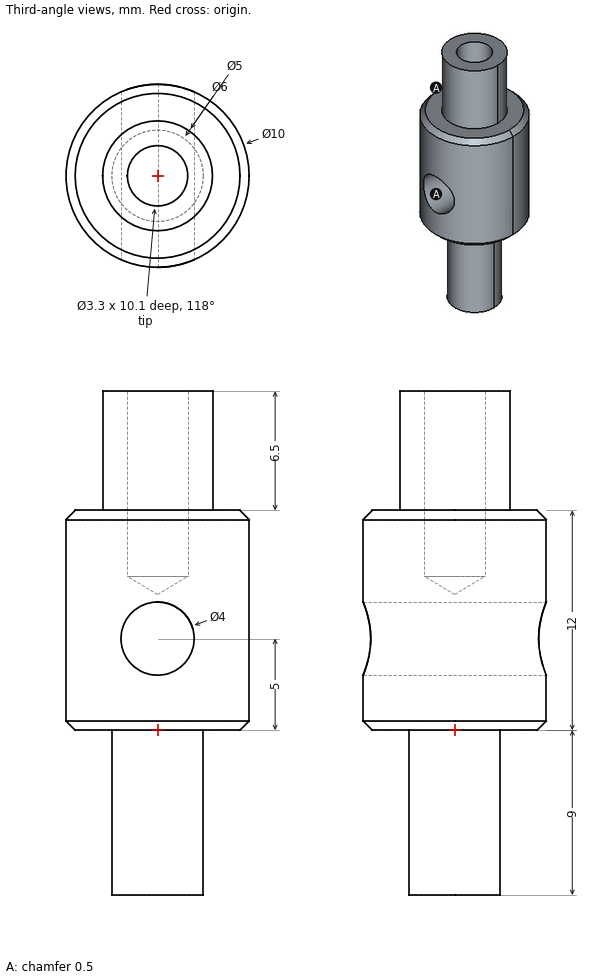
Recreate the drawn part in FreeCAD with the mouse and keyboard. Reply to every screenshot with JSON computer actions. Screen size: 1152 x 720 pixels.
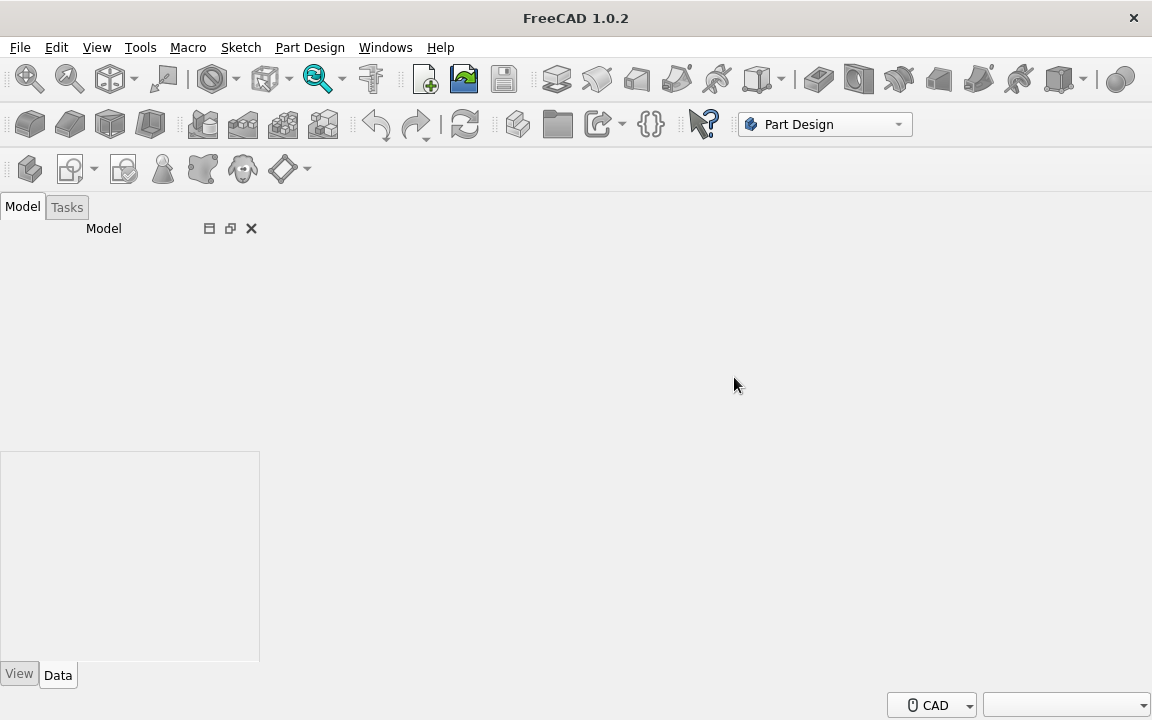
{"action": "key", "text": "ctrl+n"}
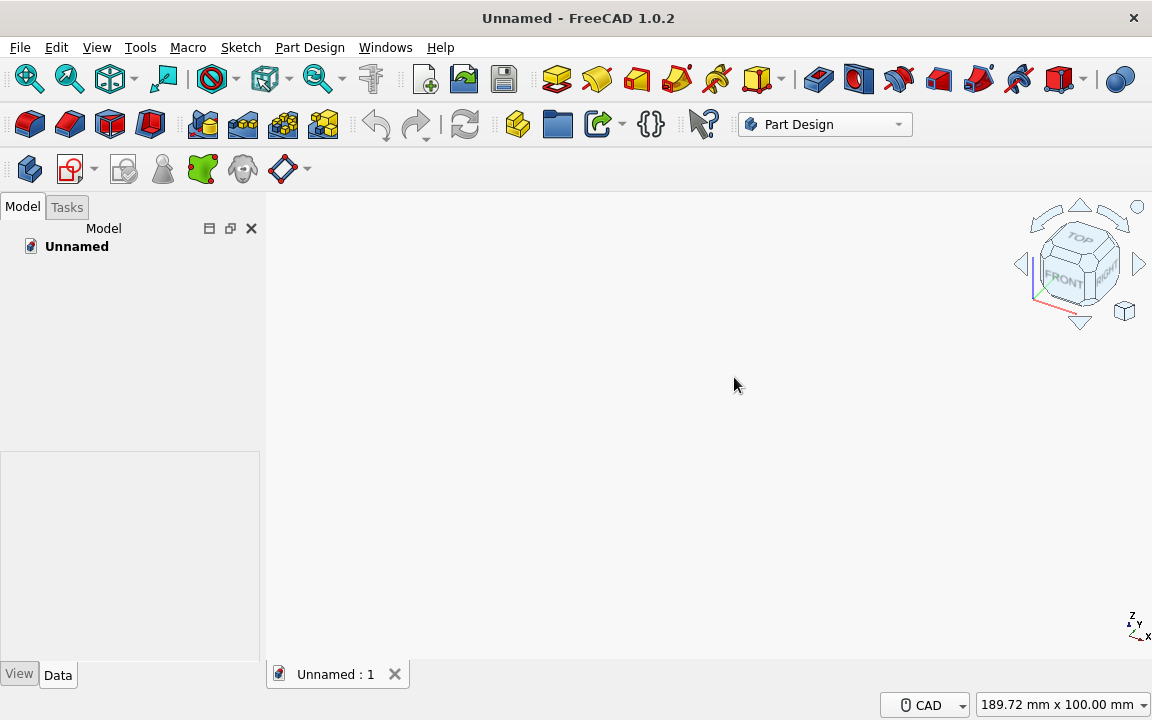
{"action": "left_click", "coordinate": [70, 170]}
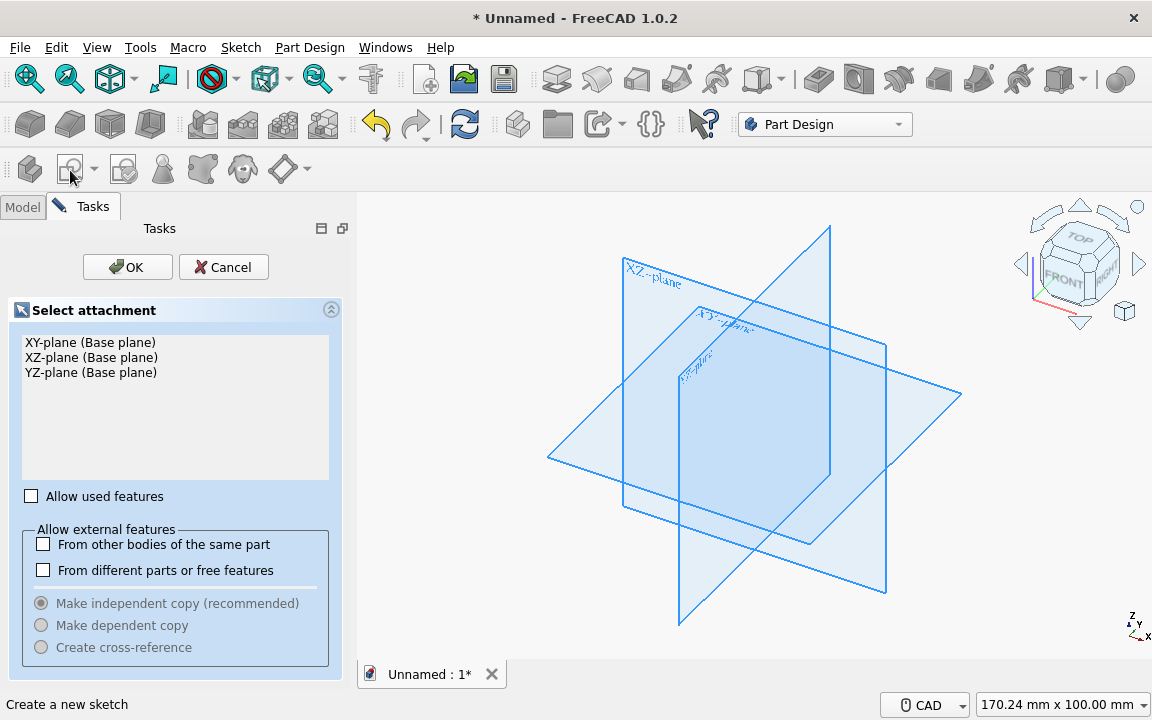
{"action": "left_click", "coordinate": [82, 342]}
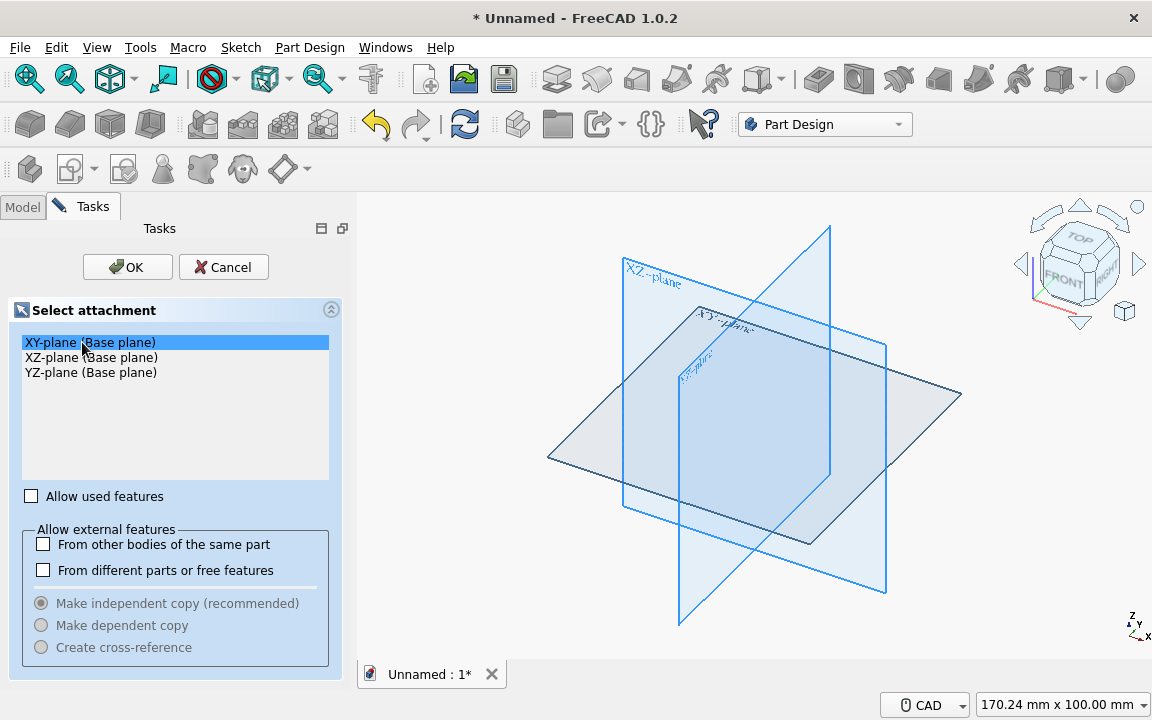
{"action": "left_click", "coordinate": [128, 267]}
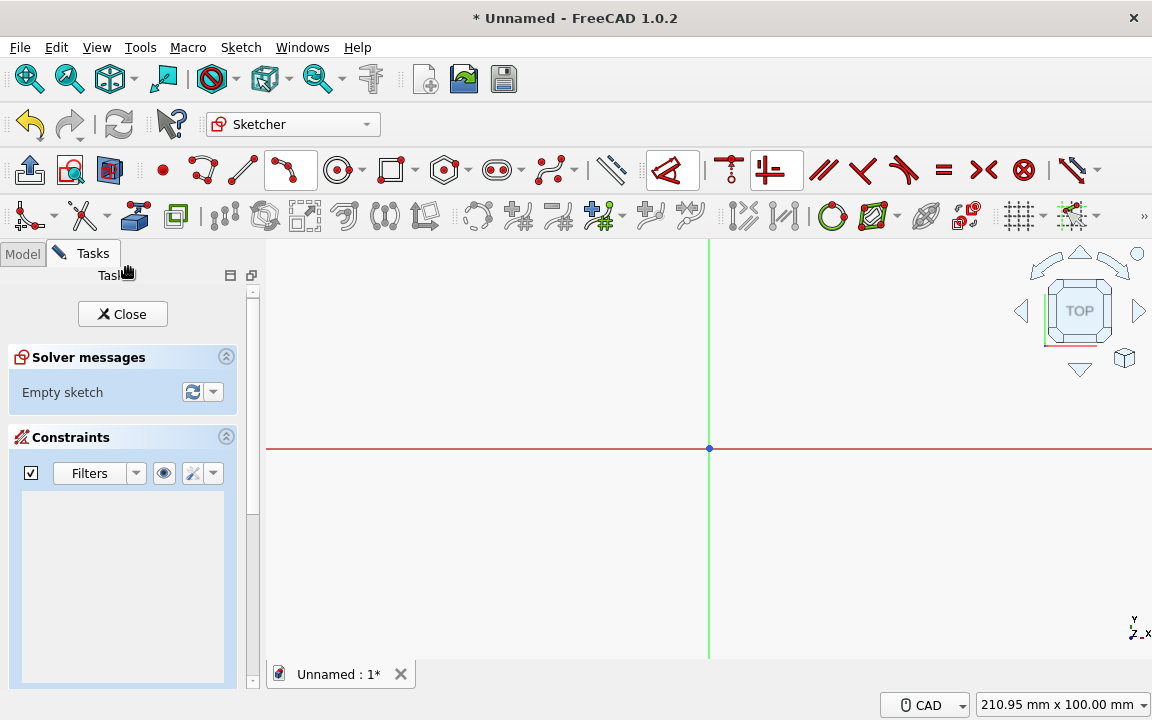
{"action": "scroll", "coordinate": [723, 449], "scroll_direction": "up", "scroll_amount": 9}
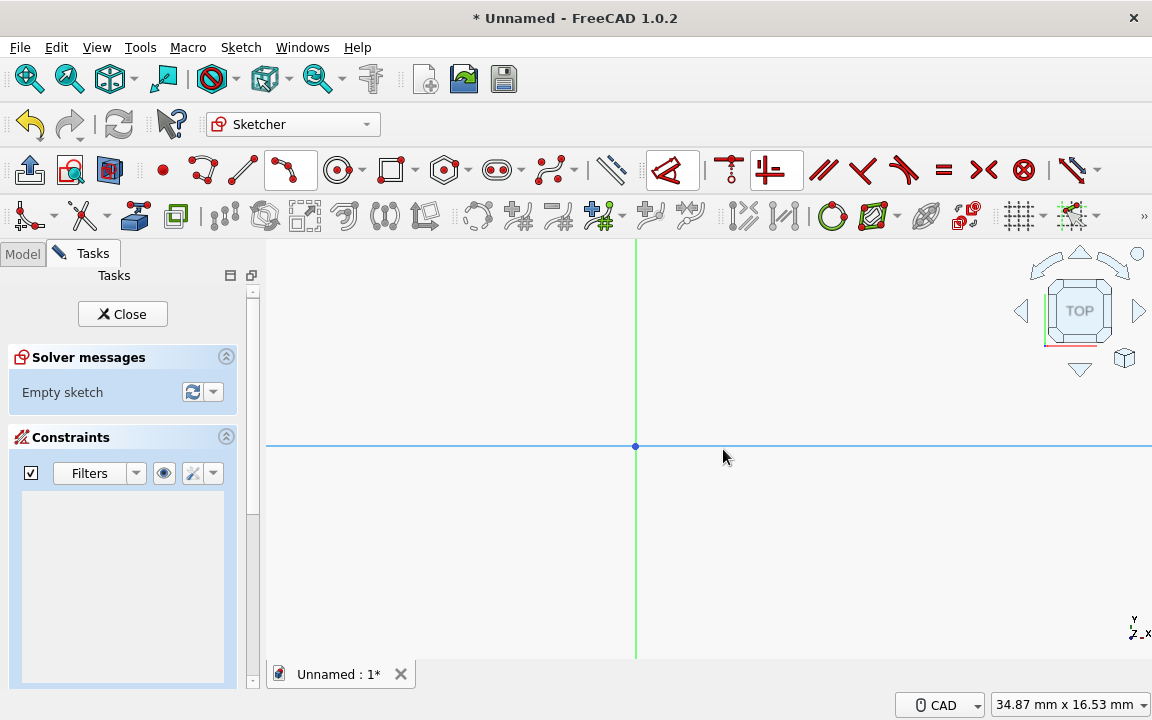
{"action": "key", "text": "g c"}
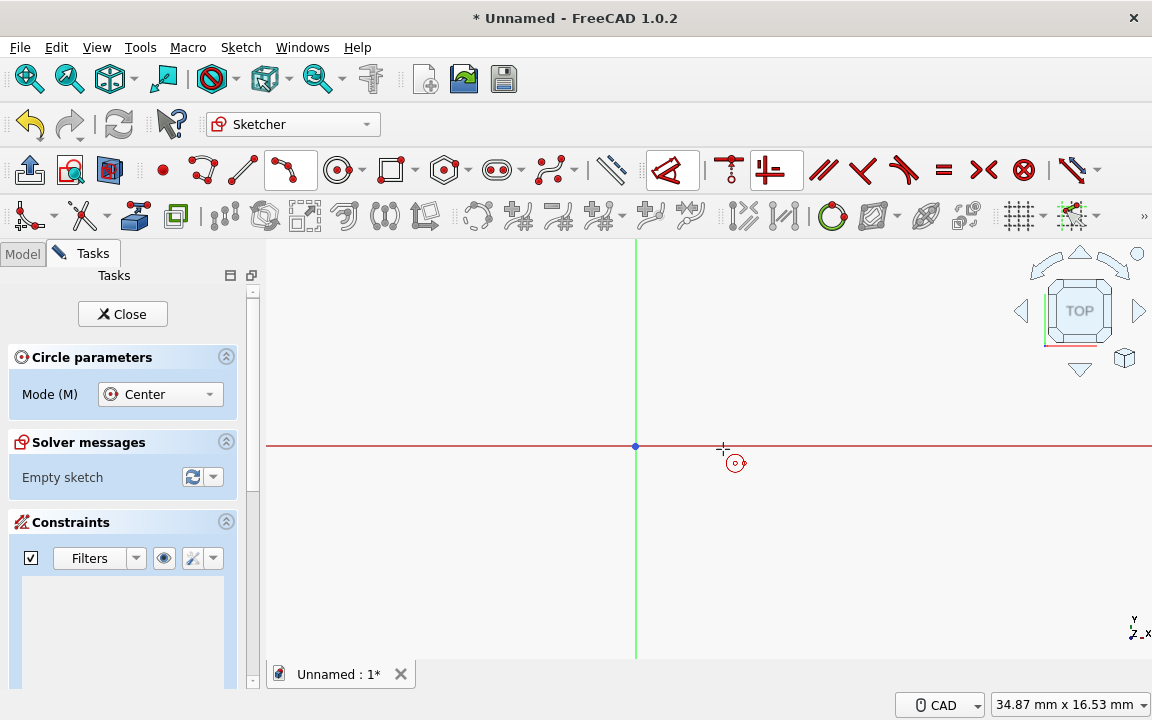
{"action": "left_click", "coordinate": [636, 446]}
{"action": "left_click", "coordinate": [726, 357]}
{"action": "key", "text": "Escape"}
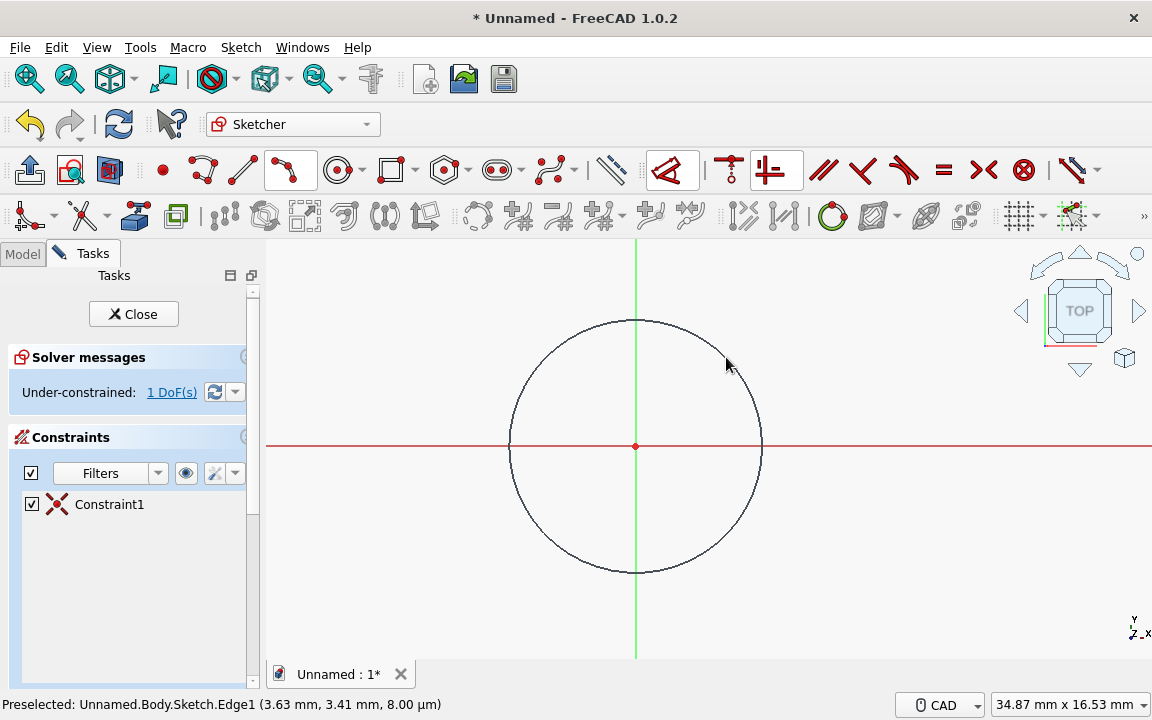
{"action": "key", "text": "d"}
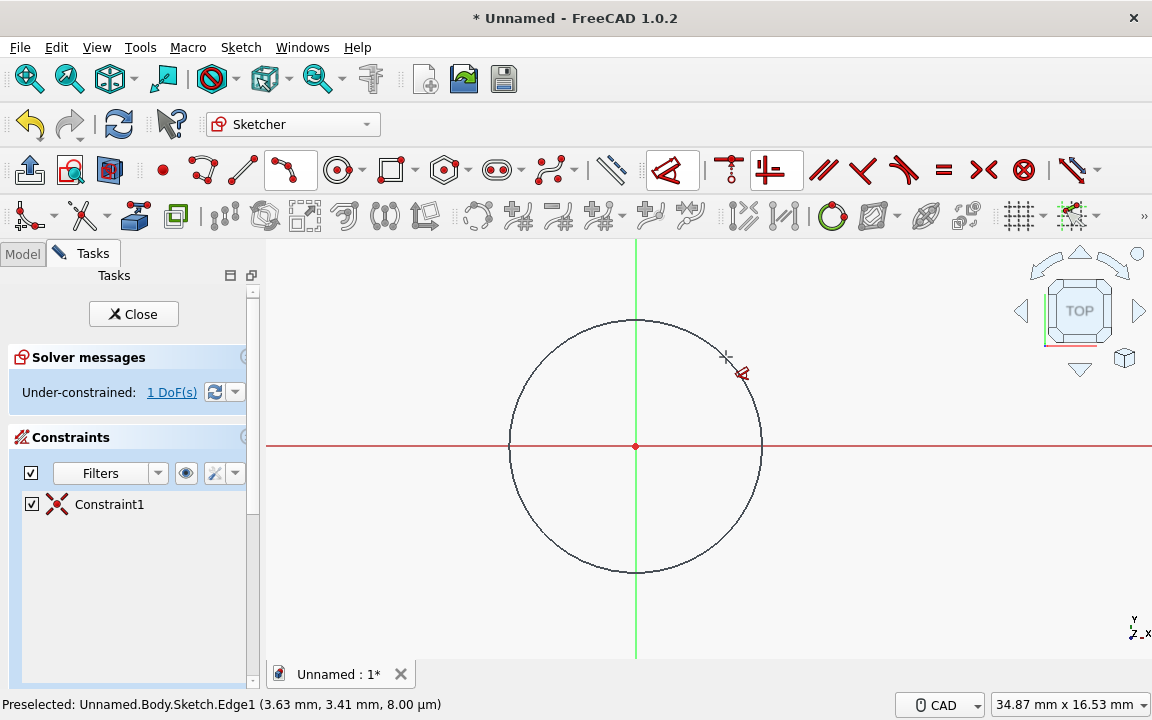
{"action": "left_click", "coordinate": [725, 357]}
{"action": "left_click", "coordinate": [748, 334]}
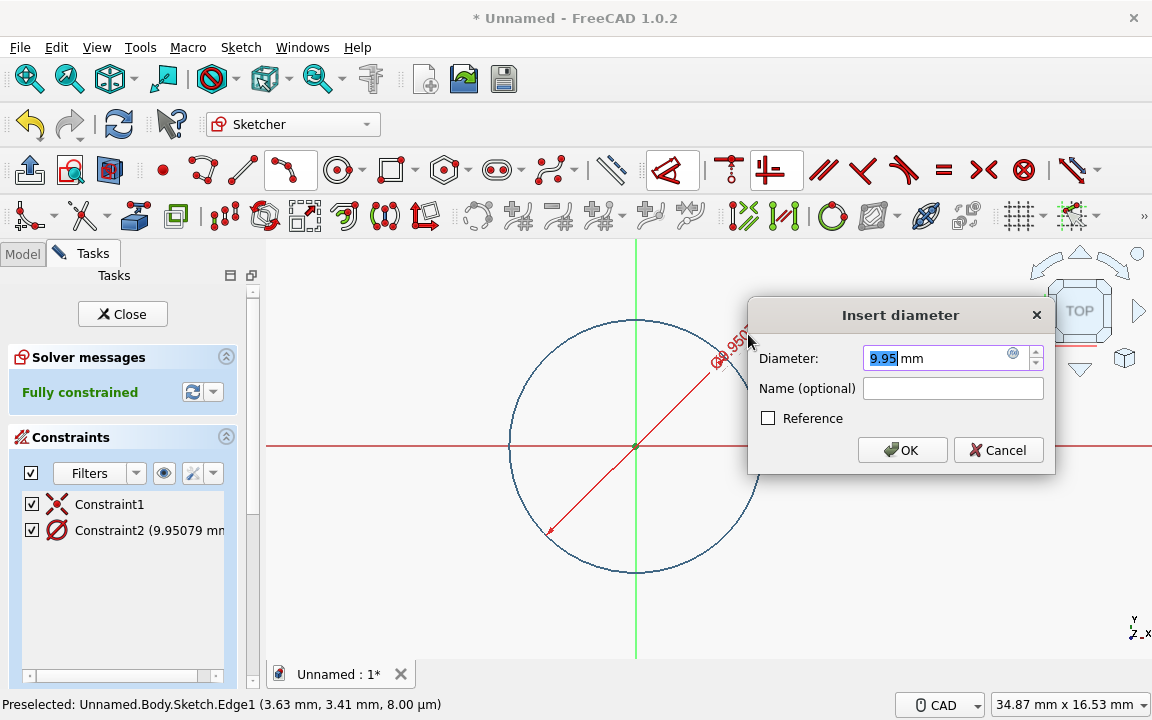
{"action": "type", "text": "10"}
{"action": "key", "text": "Return"}
{"action": "key", "text": "Escape"}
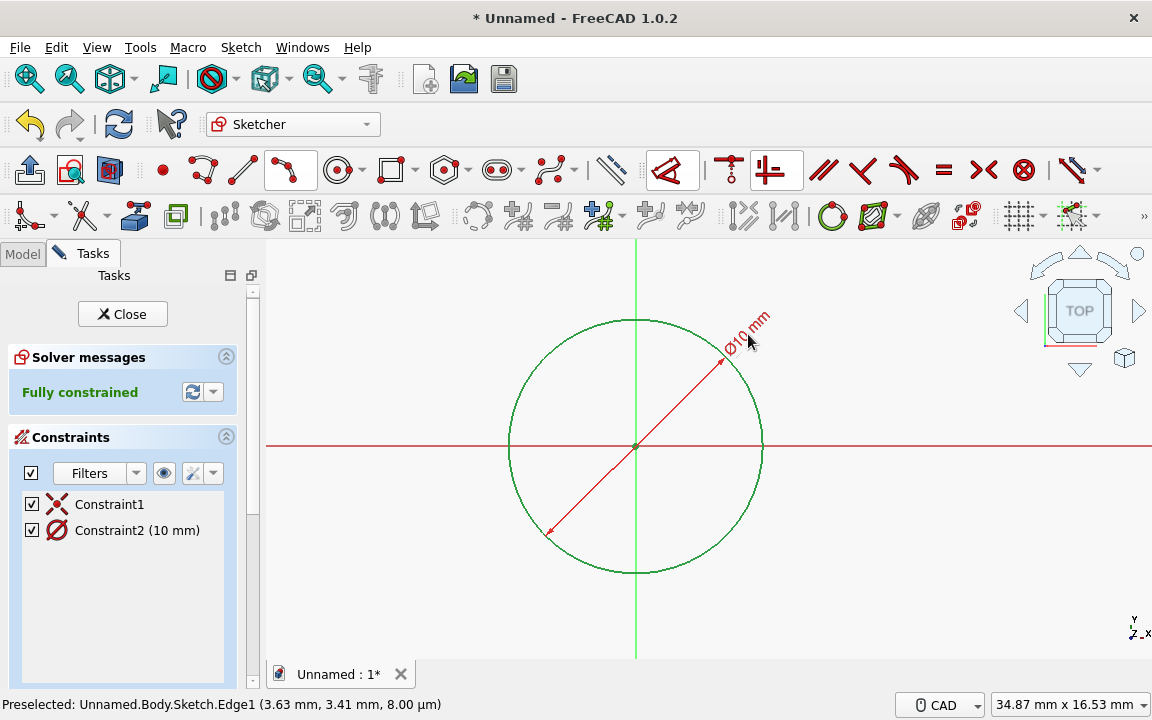
{"action": "left_click", "coordinate": [123, 314]}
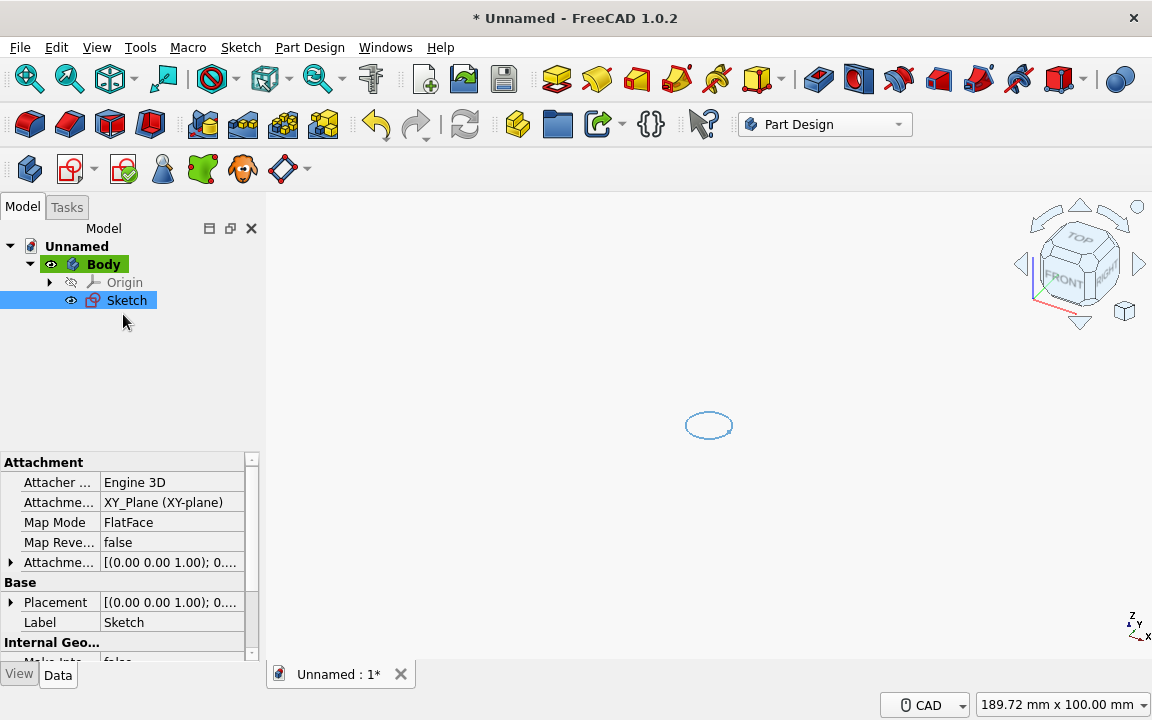
{"action": "left_click", "coordinate": [558, 80]}